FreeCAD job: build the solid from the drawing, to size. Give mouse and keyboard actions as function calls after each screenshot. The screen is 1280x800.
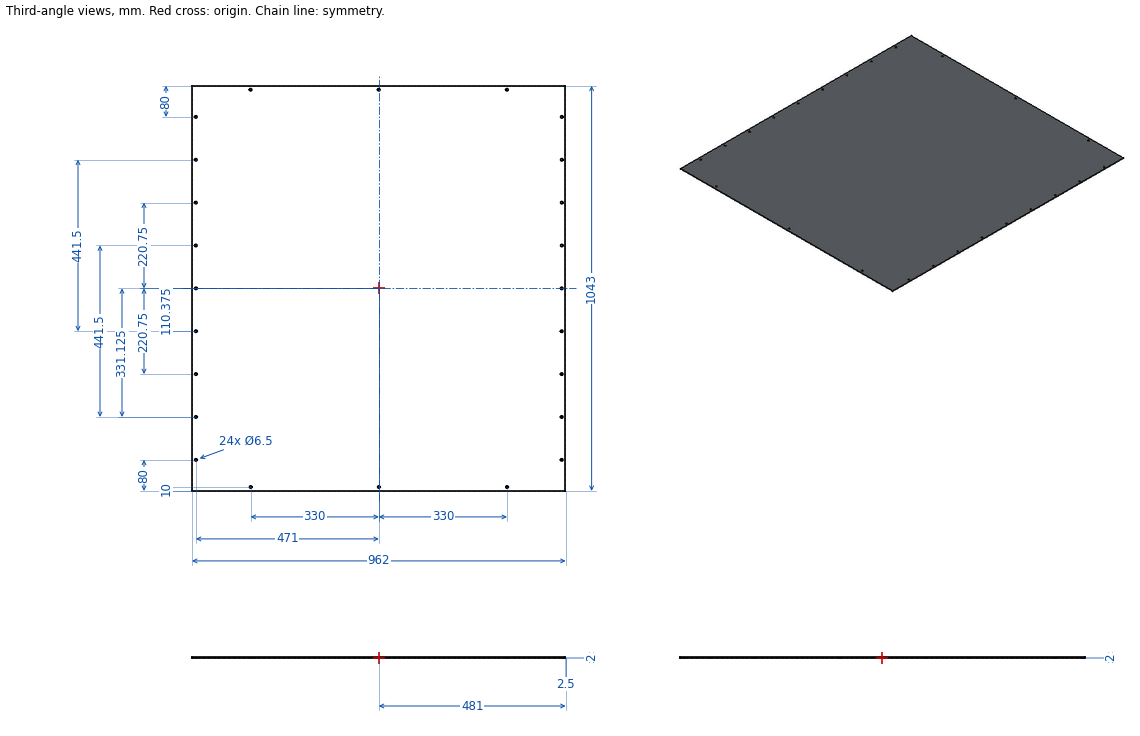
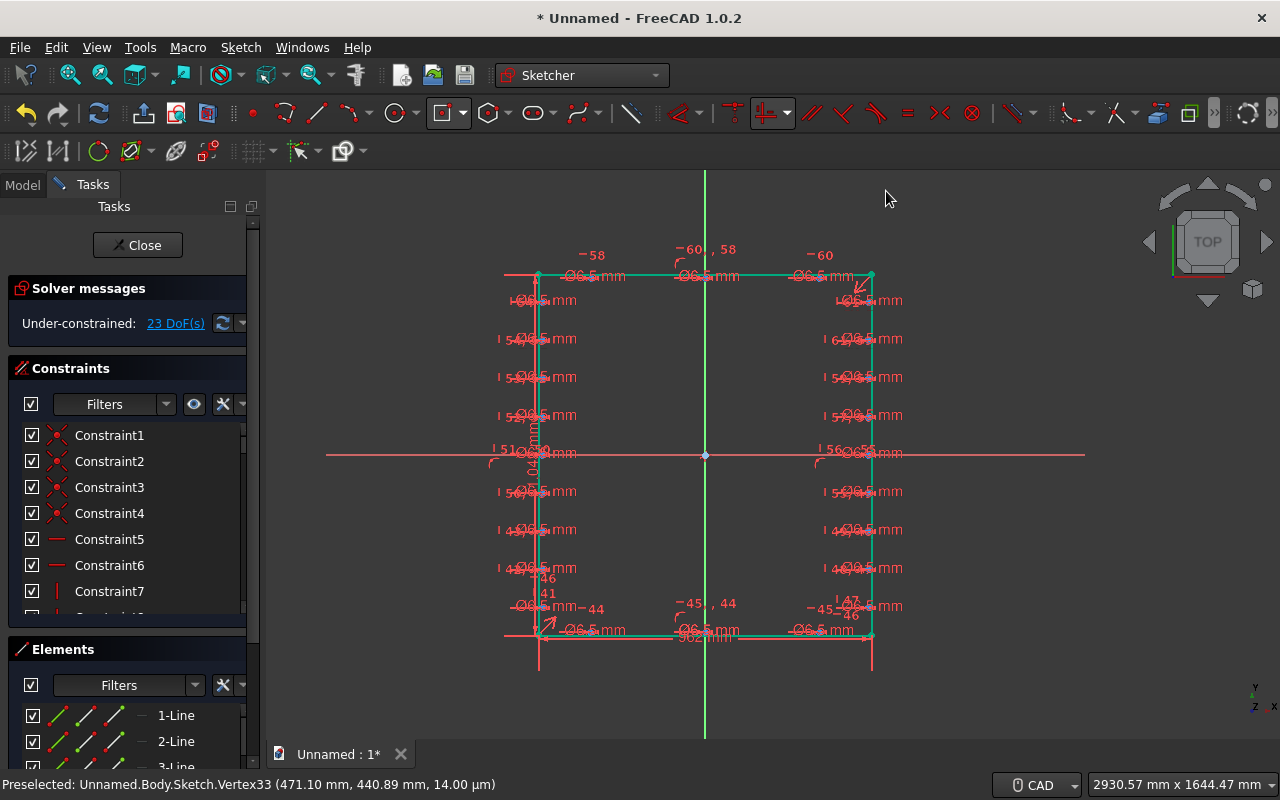
click(542, 570)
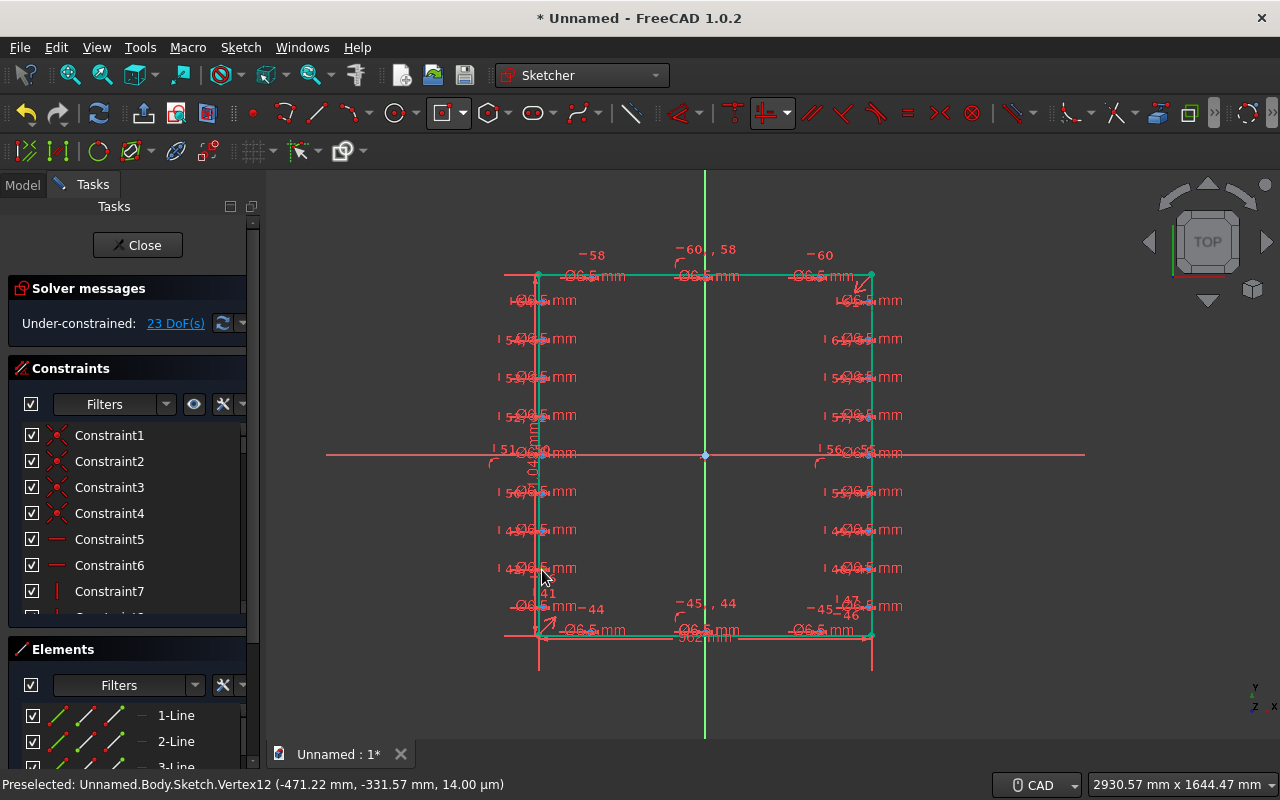
click(868, 570)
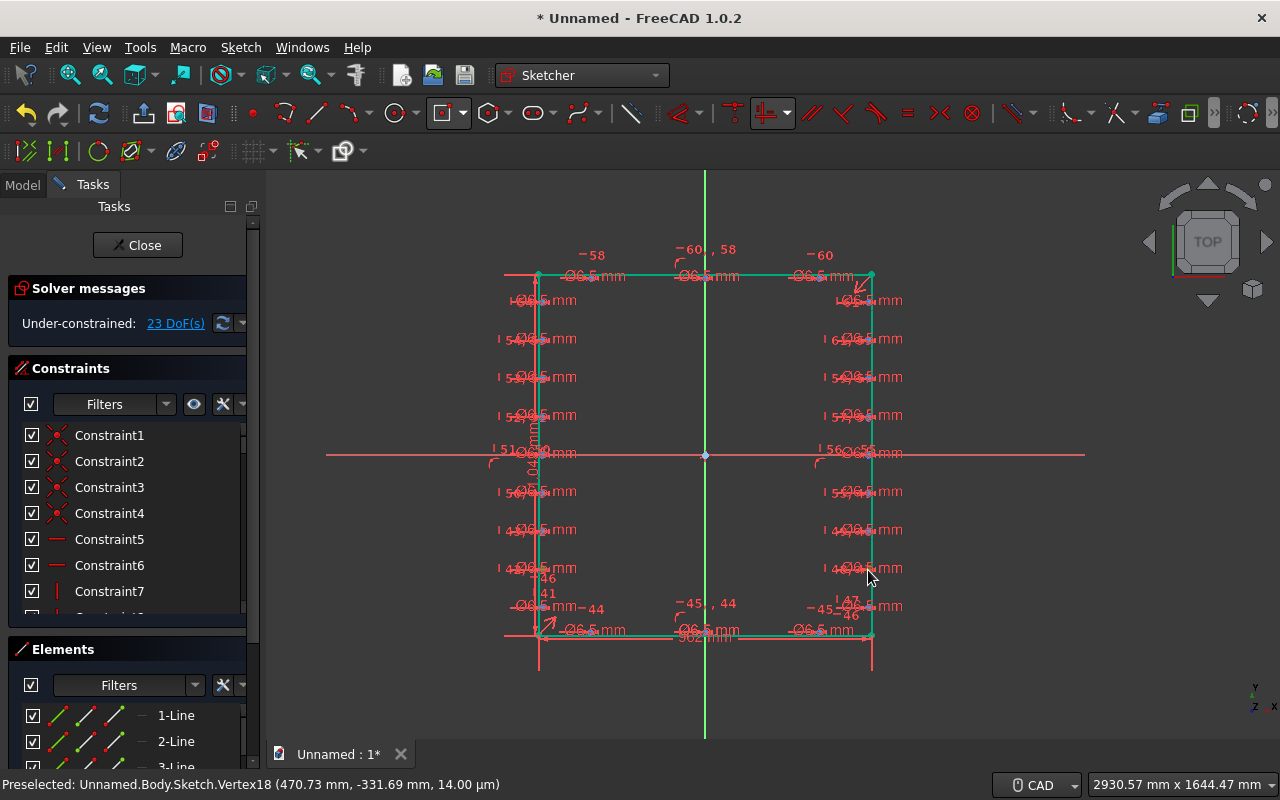
click(705, 674)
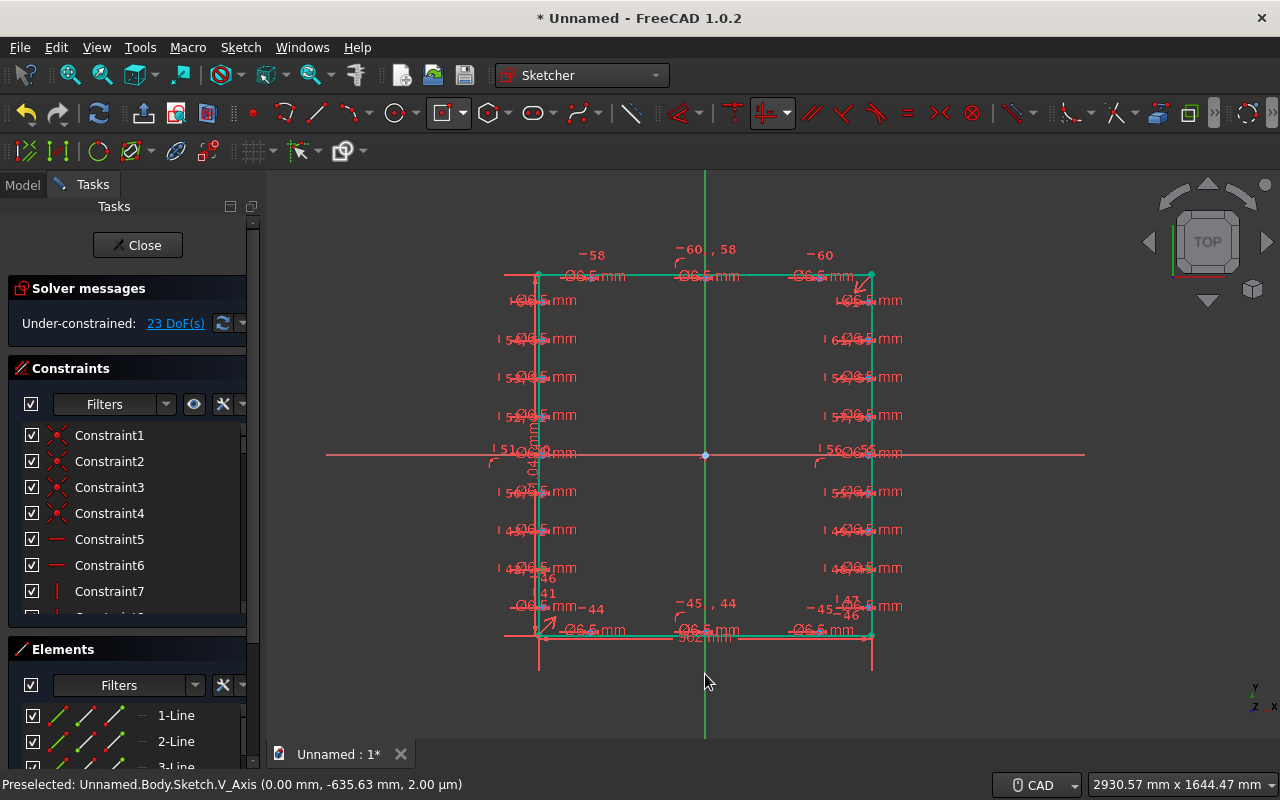
click(940, 114)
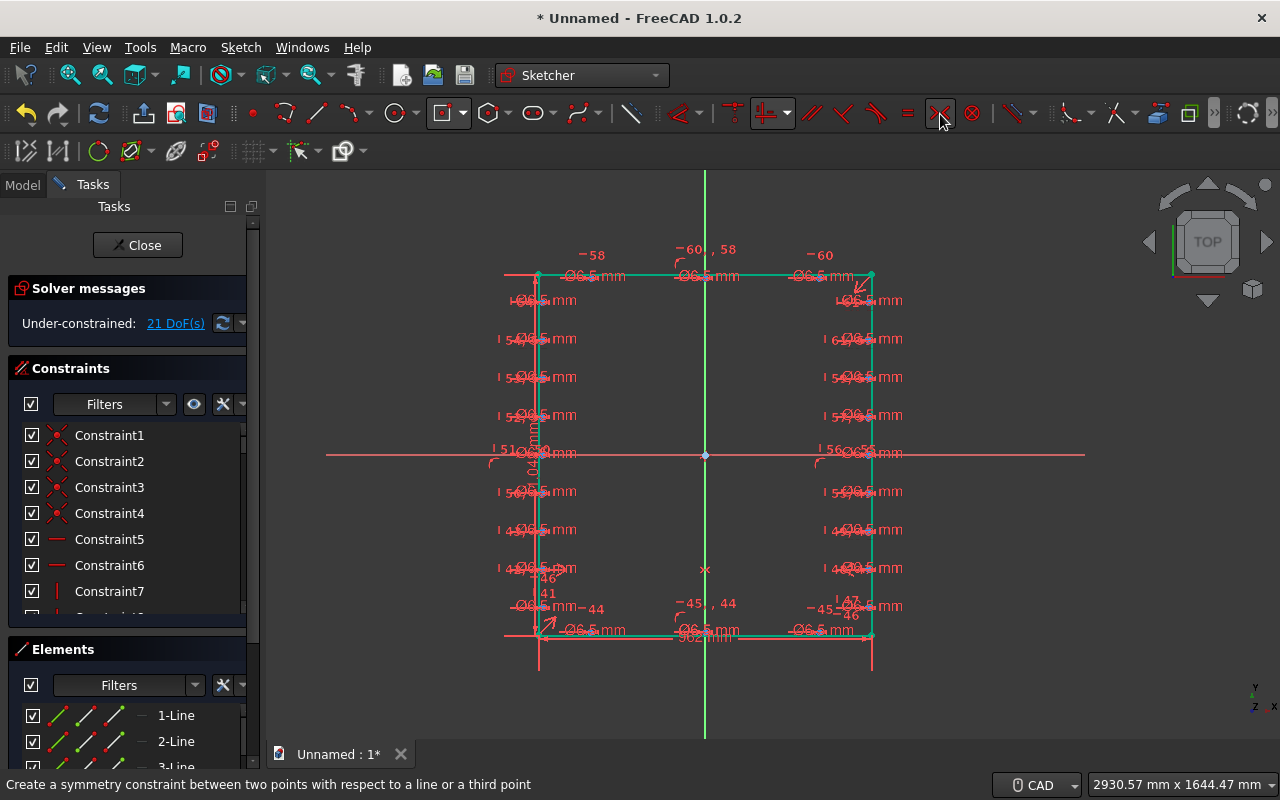
click(591, 632)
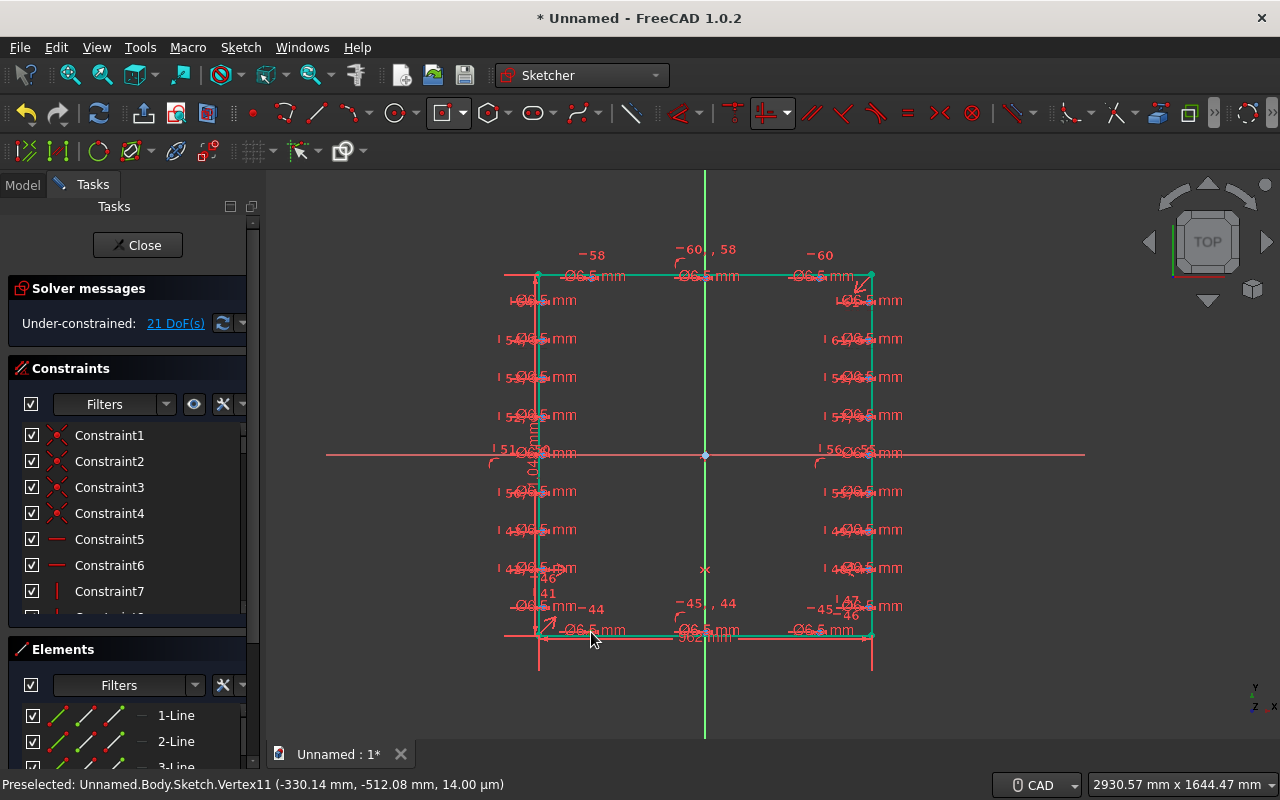
click(591, 278)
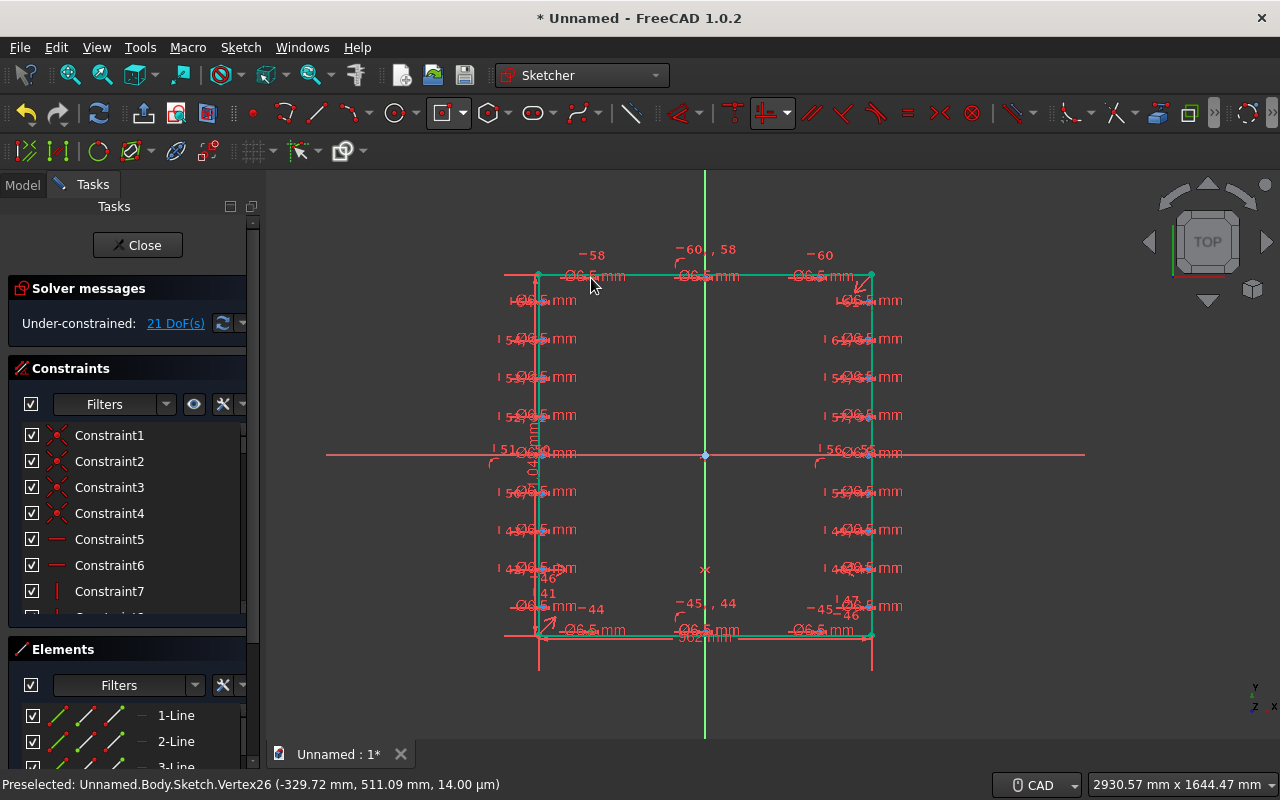
click(353, 455)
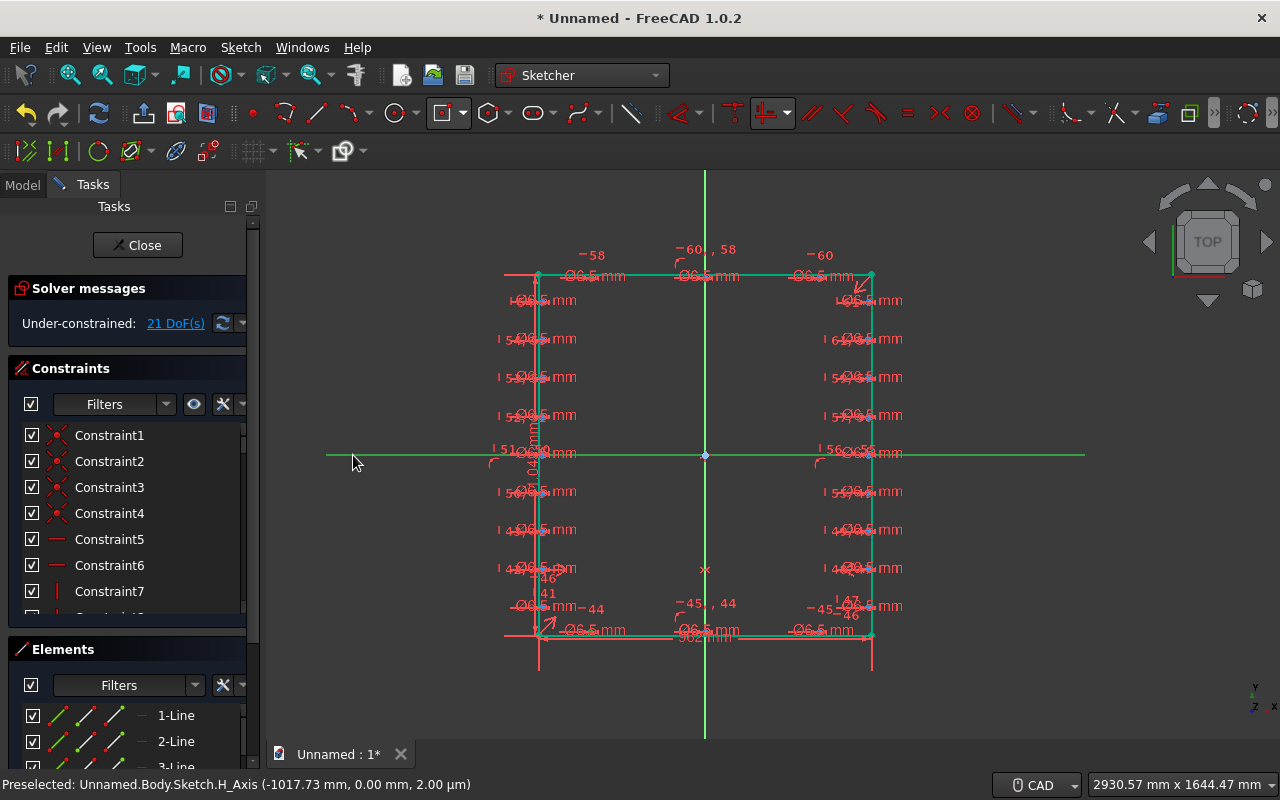
click(940, 114)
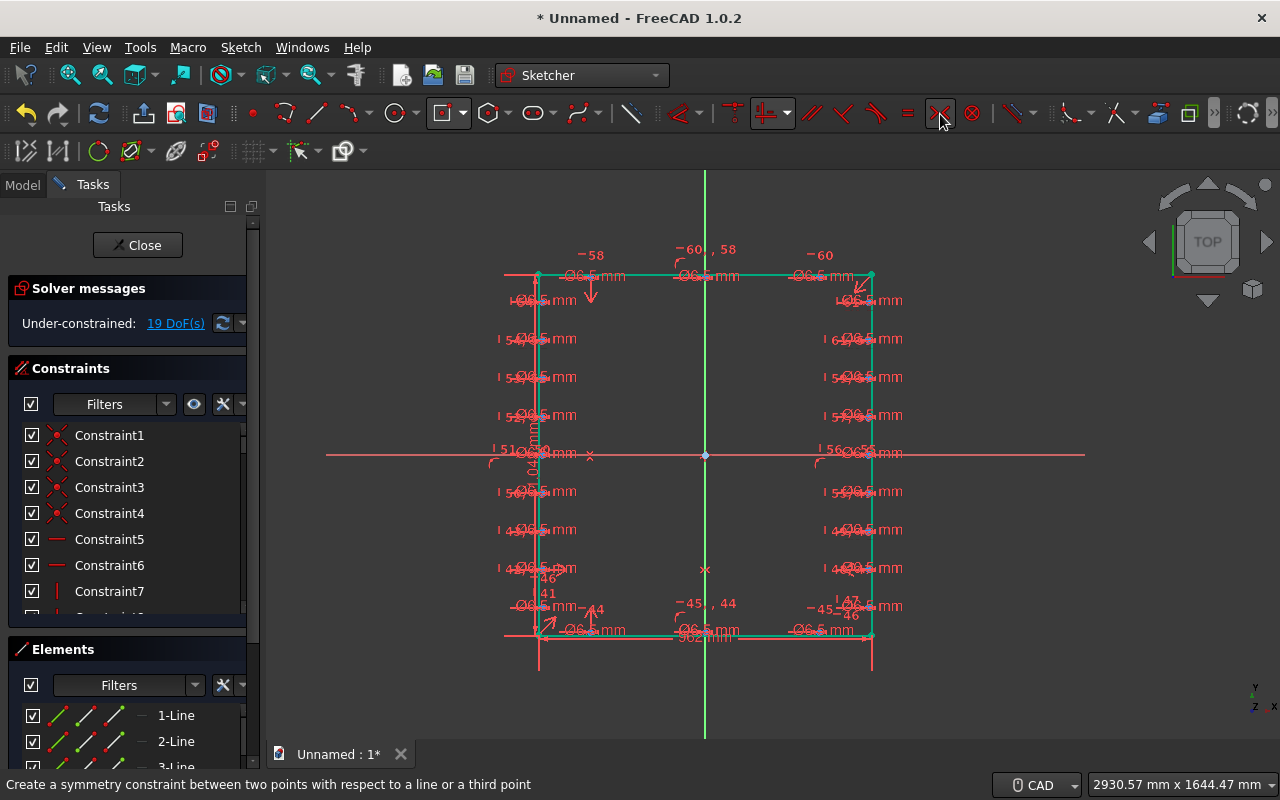
key(d)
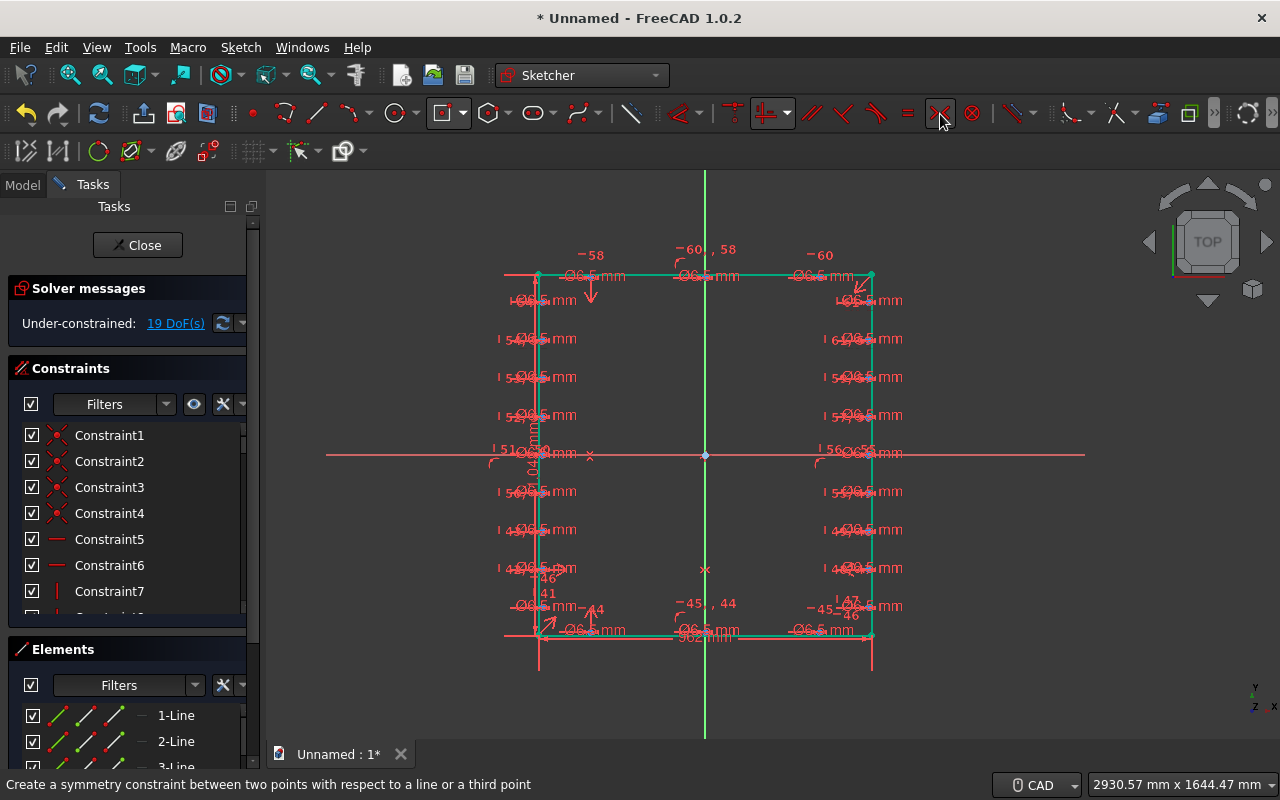
click(542, 608)
click(624, 421)